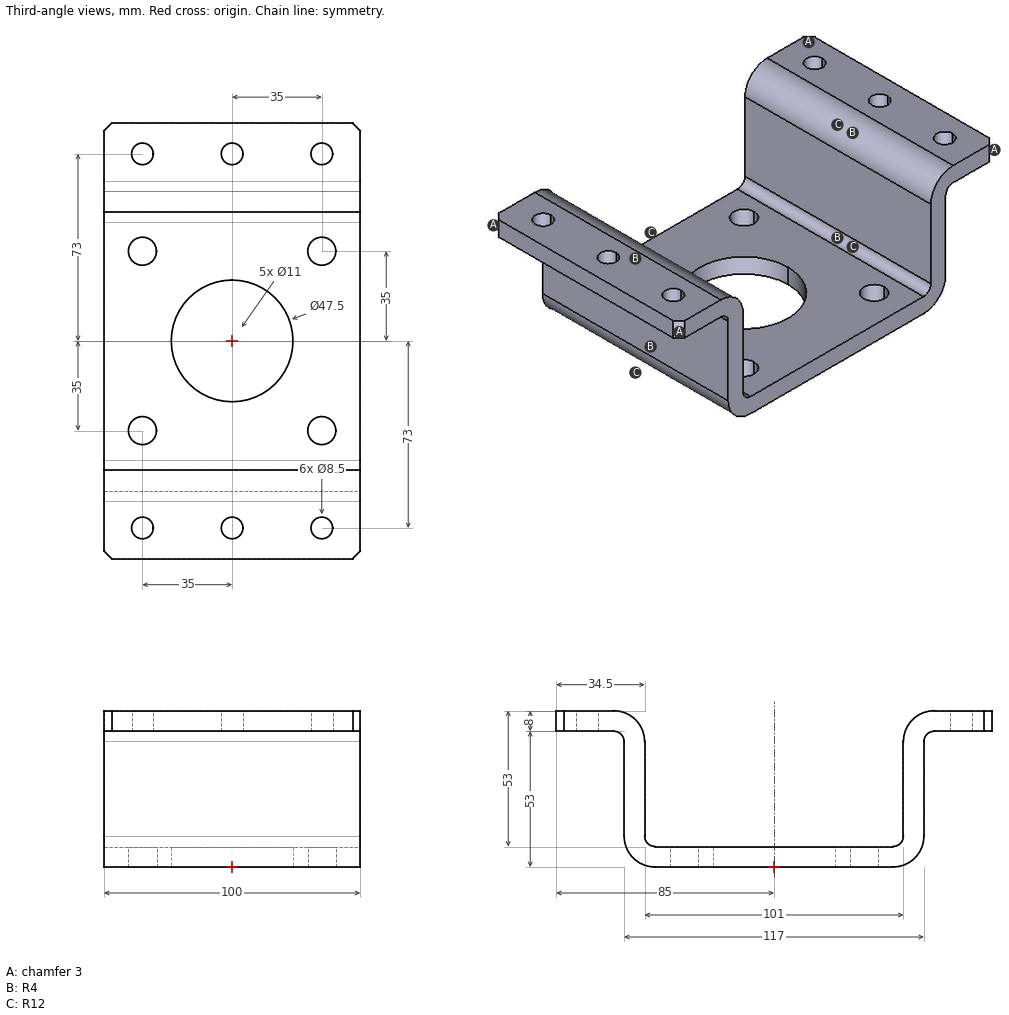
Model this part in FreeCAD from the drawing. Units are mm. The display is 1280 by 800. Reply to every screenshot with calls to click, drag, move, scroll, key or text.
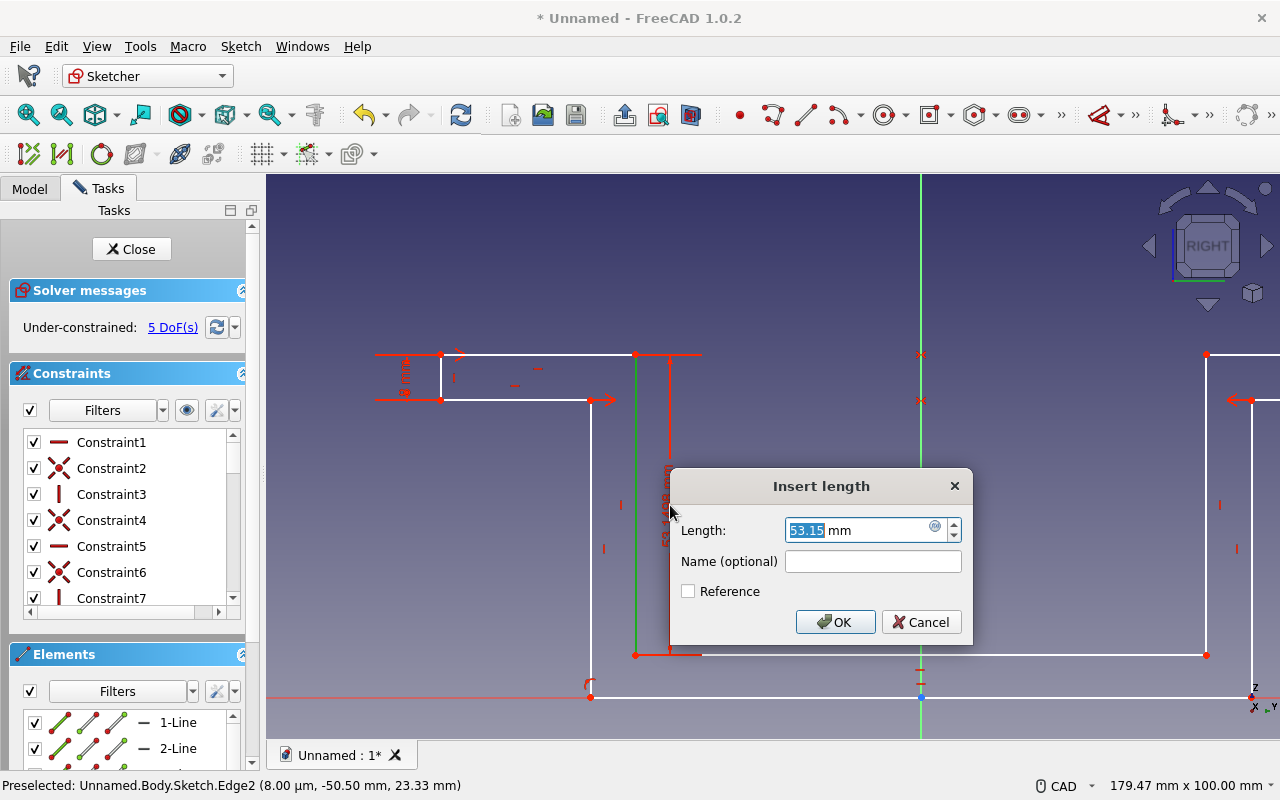
text(53)
key(Return)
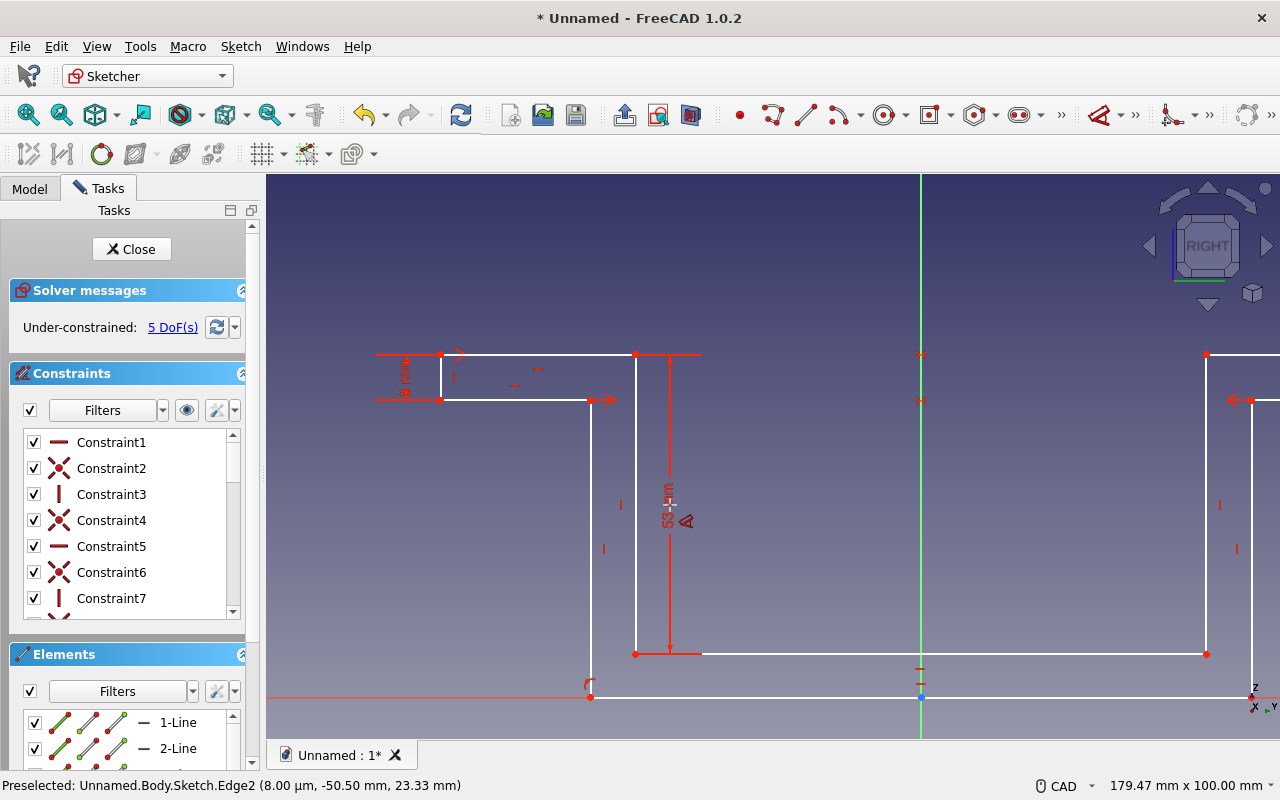
click(591, 489)
click(557, 549)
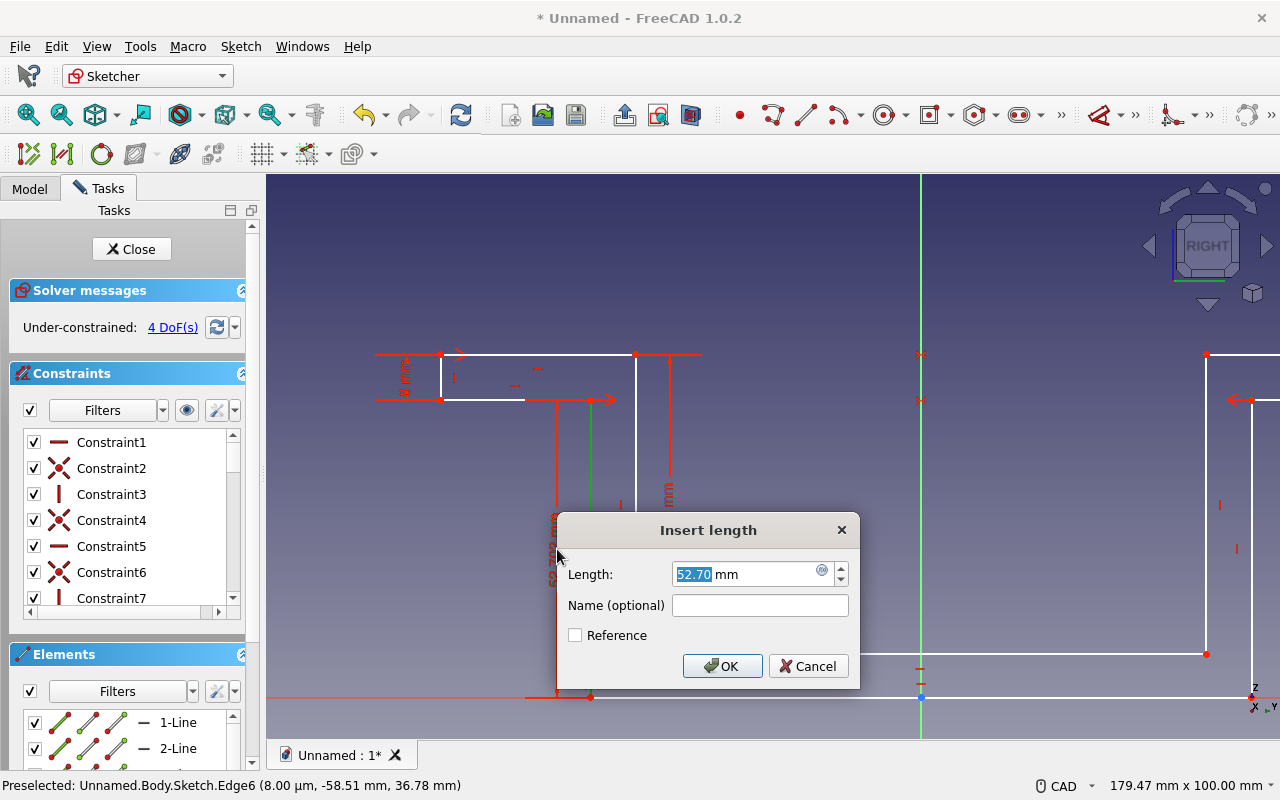
text(53)
key(Return)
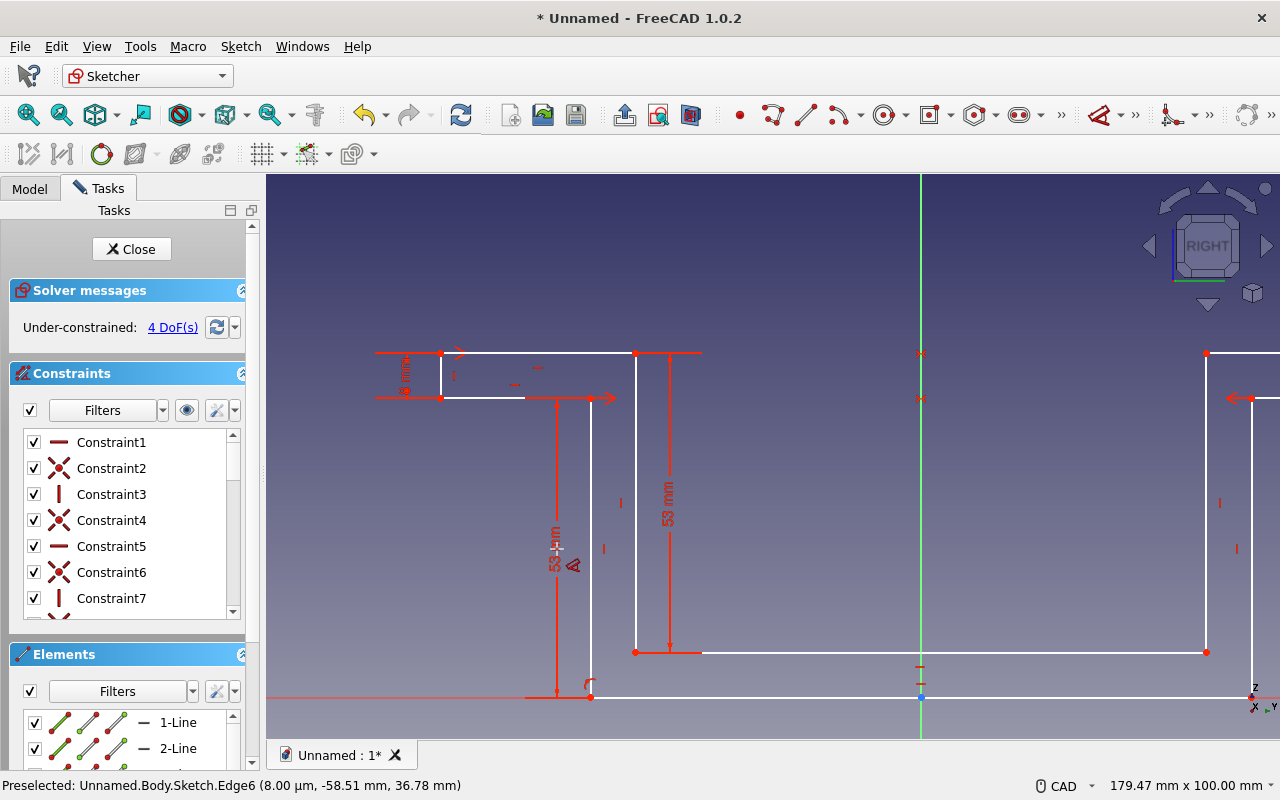
click(1035, 653)
click(875, 619)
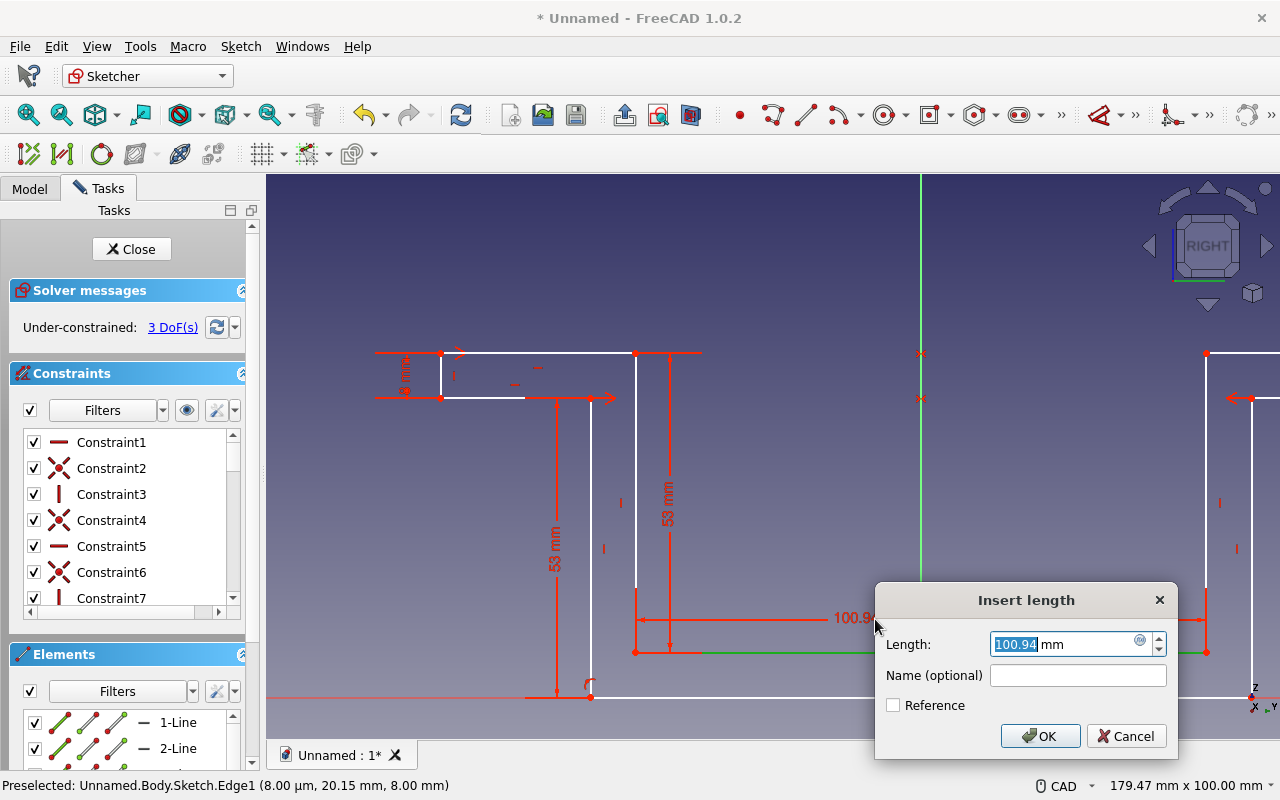
text(101)
key(Return)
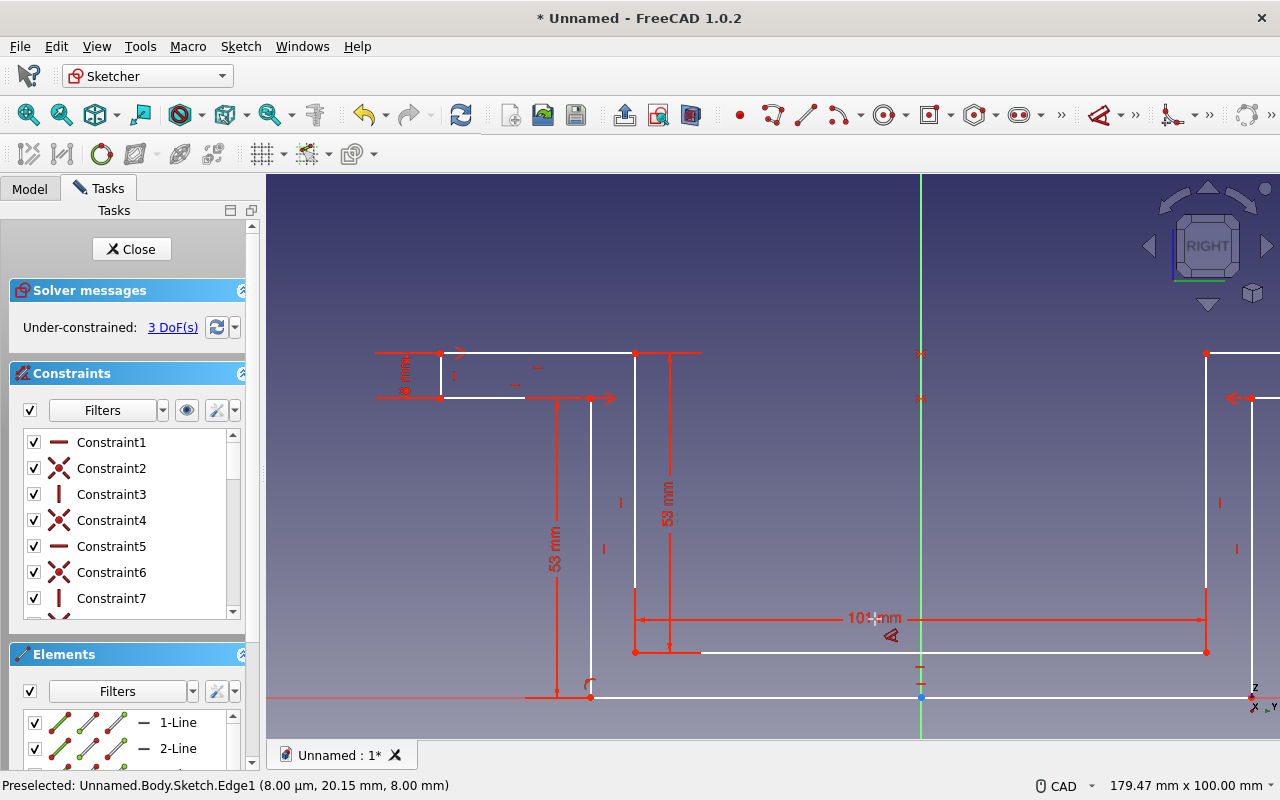
click(789, 698)
click(732, 616)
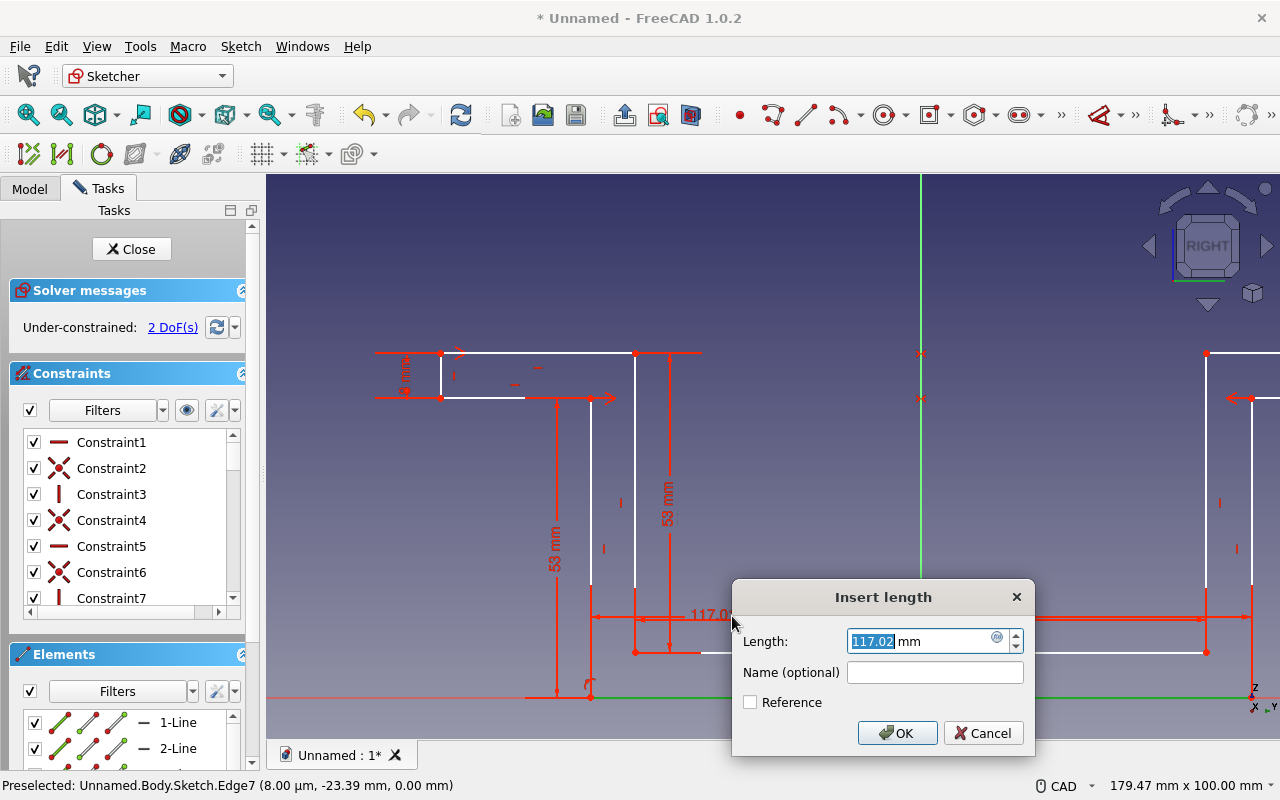
text(117)
key(Return)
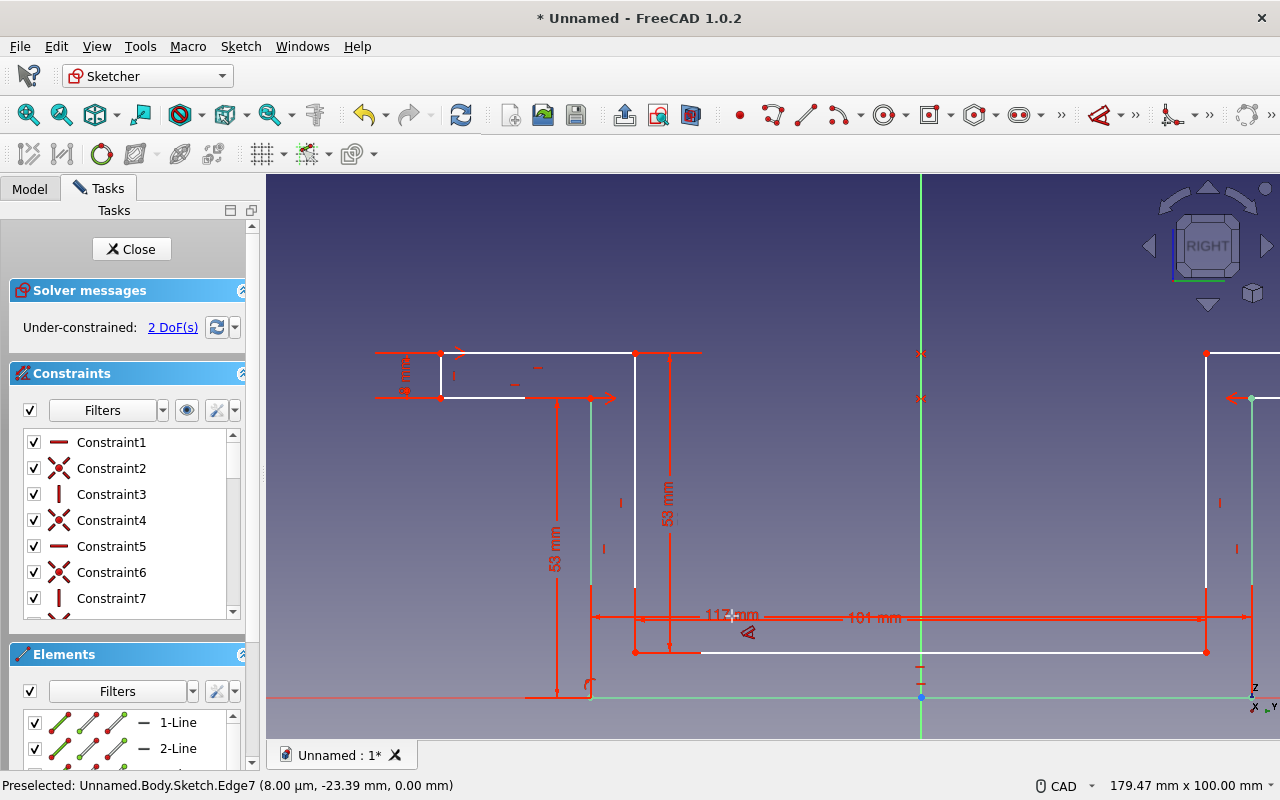
click(441, 353)
click(681, 319)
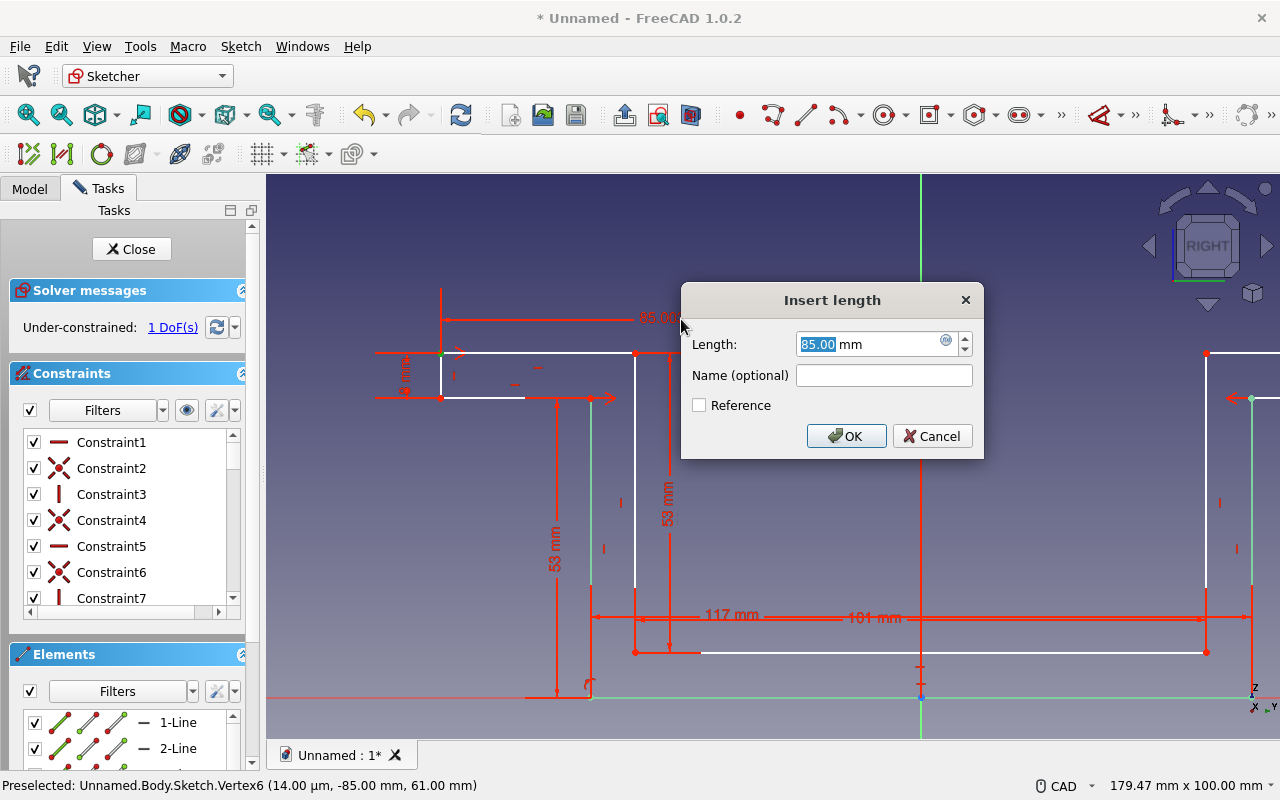
text(85)
key(Return)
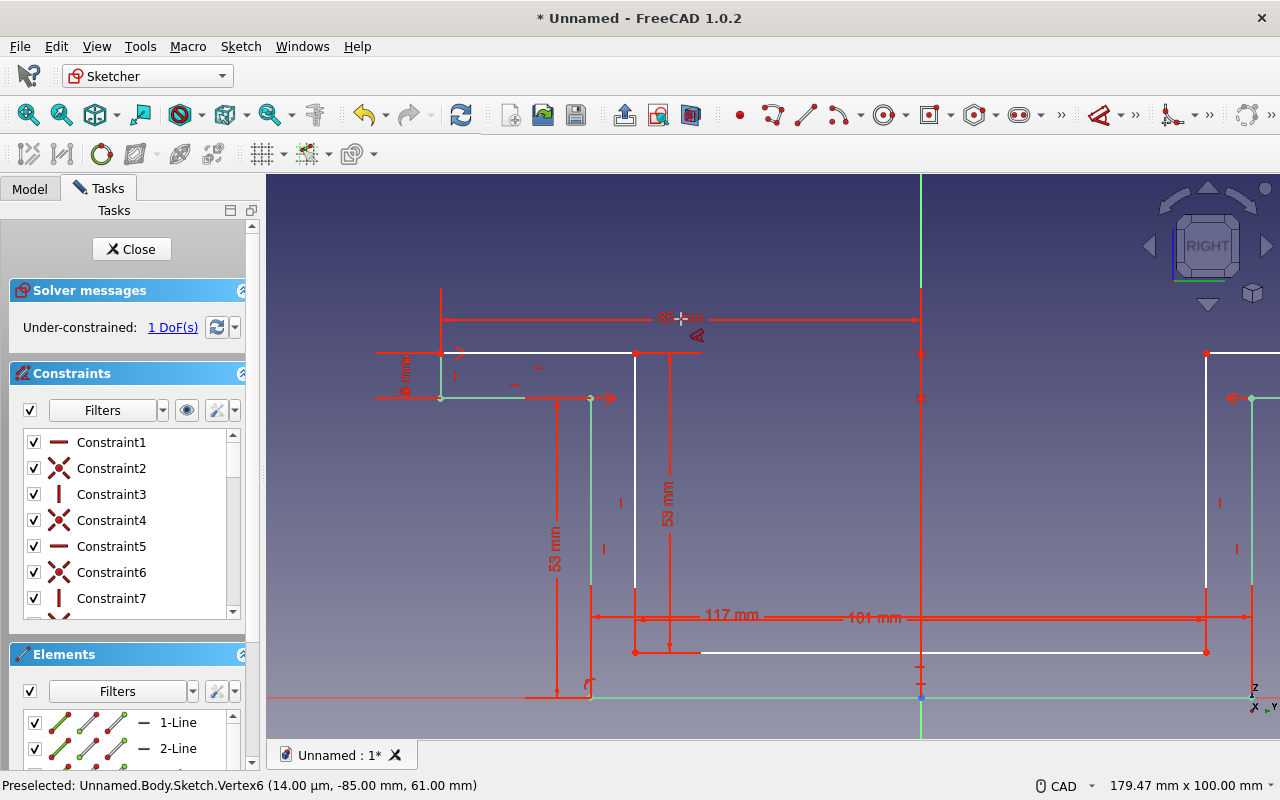
click(577, 353)
click(538, 319)